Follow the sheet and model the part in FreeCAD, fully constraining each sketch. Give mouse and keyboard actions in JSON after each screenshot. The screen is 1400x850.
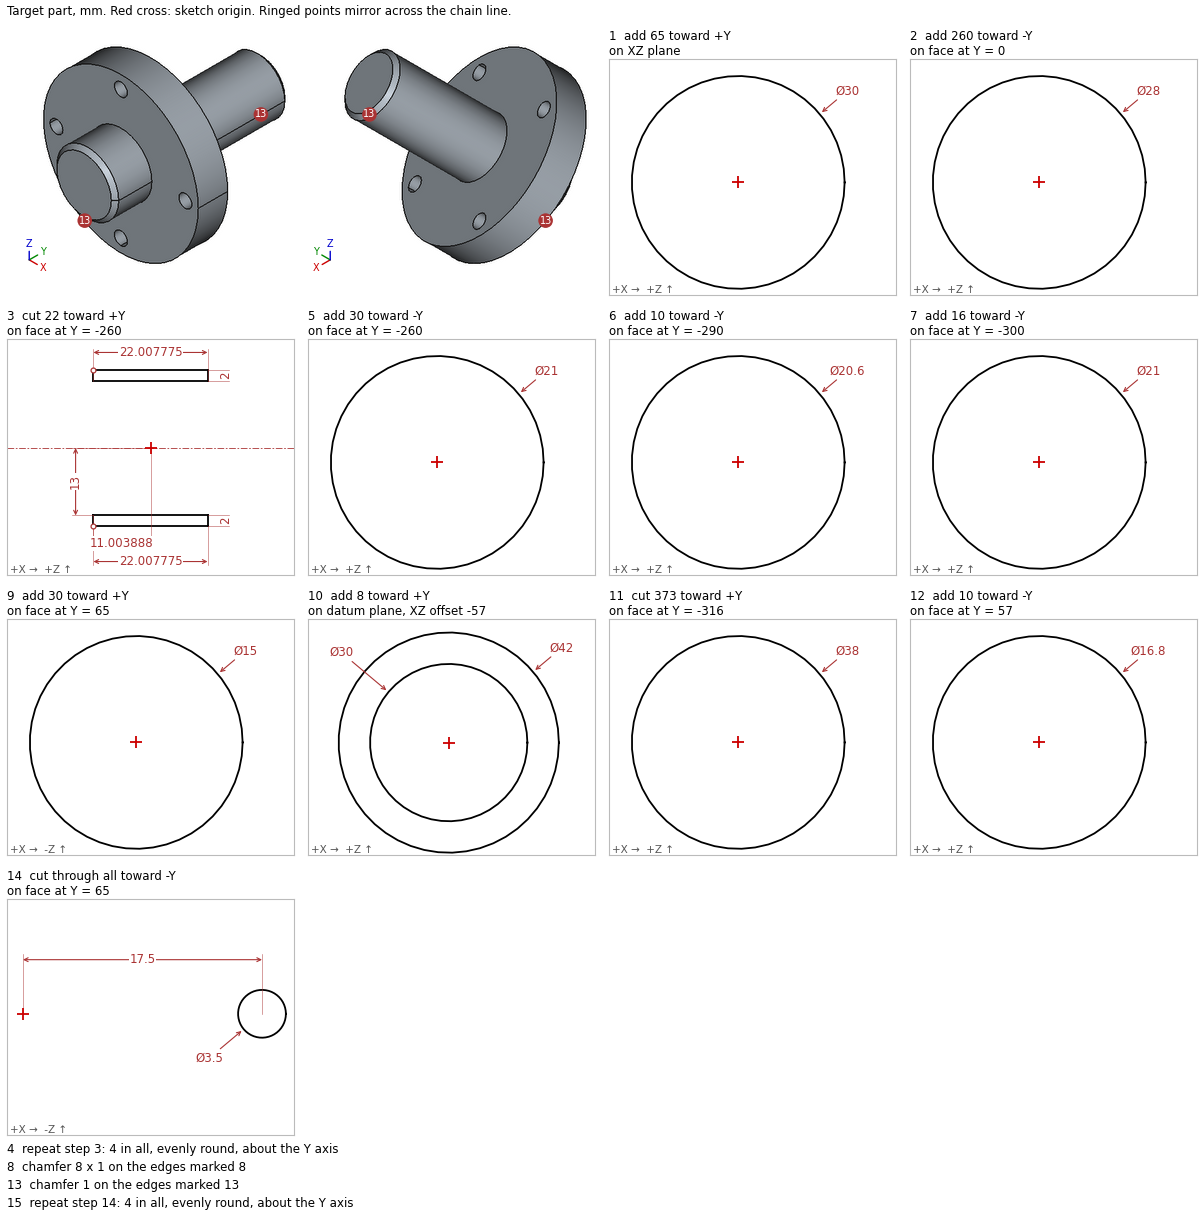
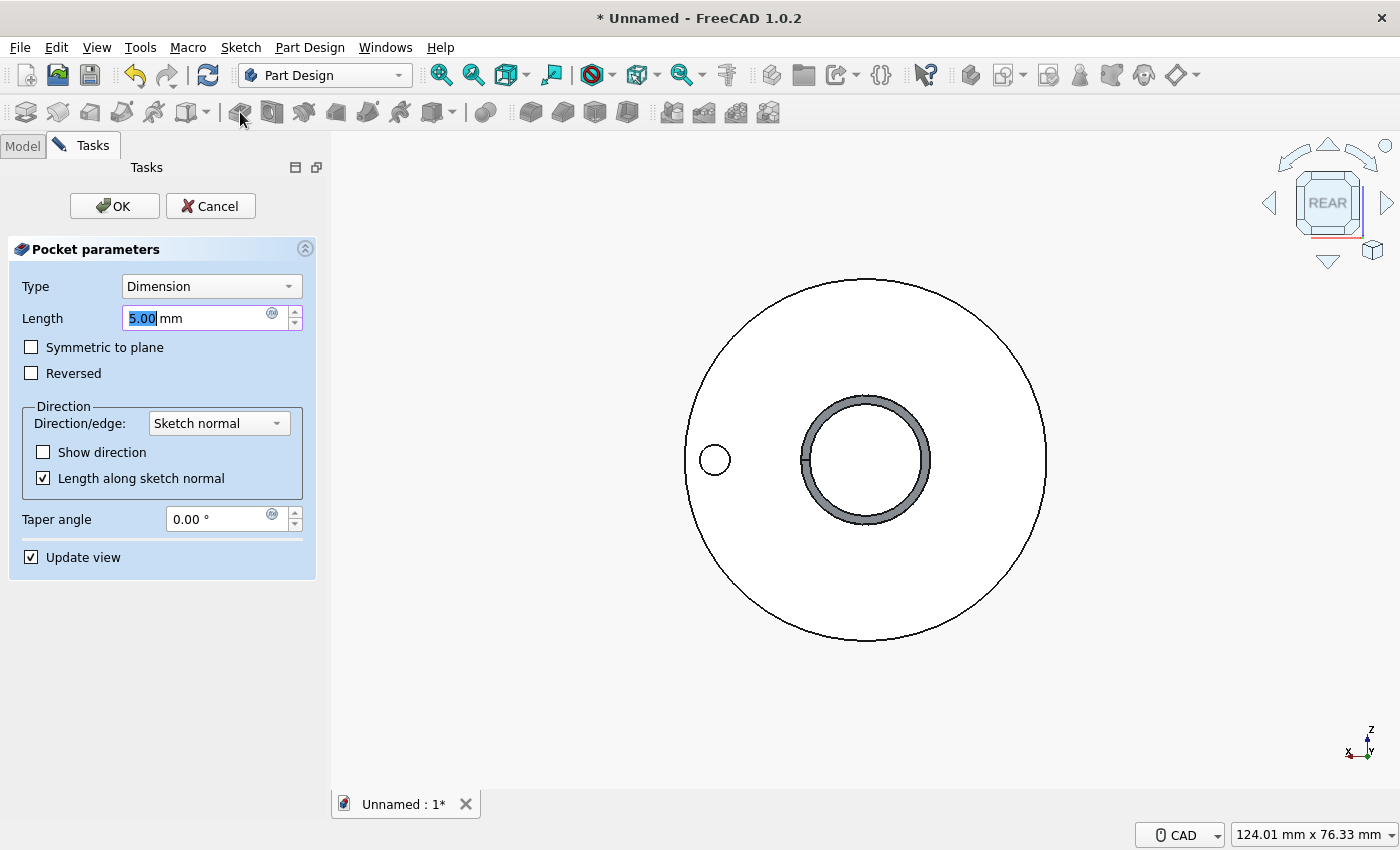
{"action": "left_click", "coordinate": [212, 286]}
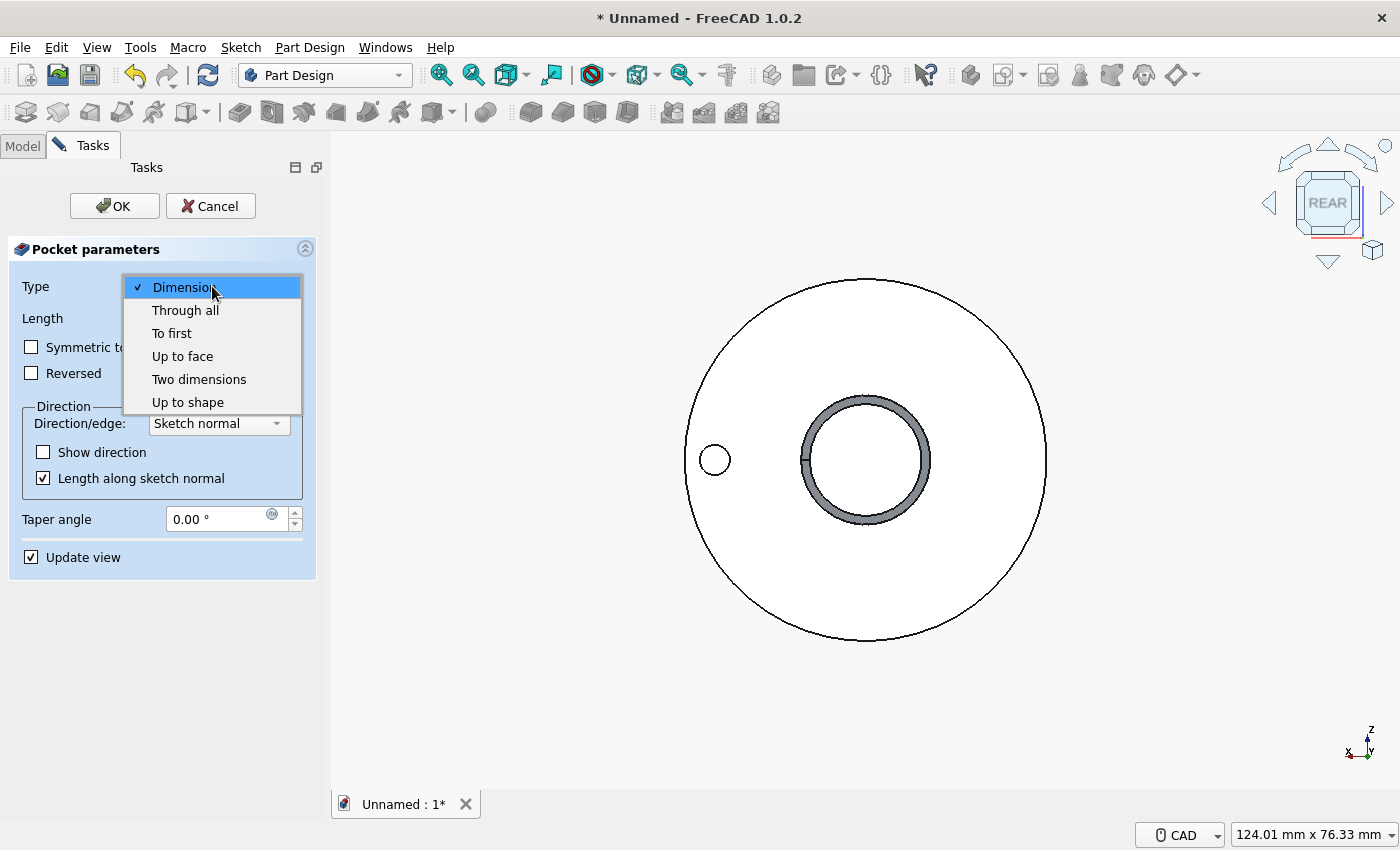
{"action": "left_click", "coordinate": [212, 310]}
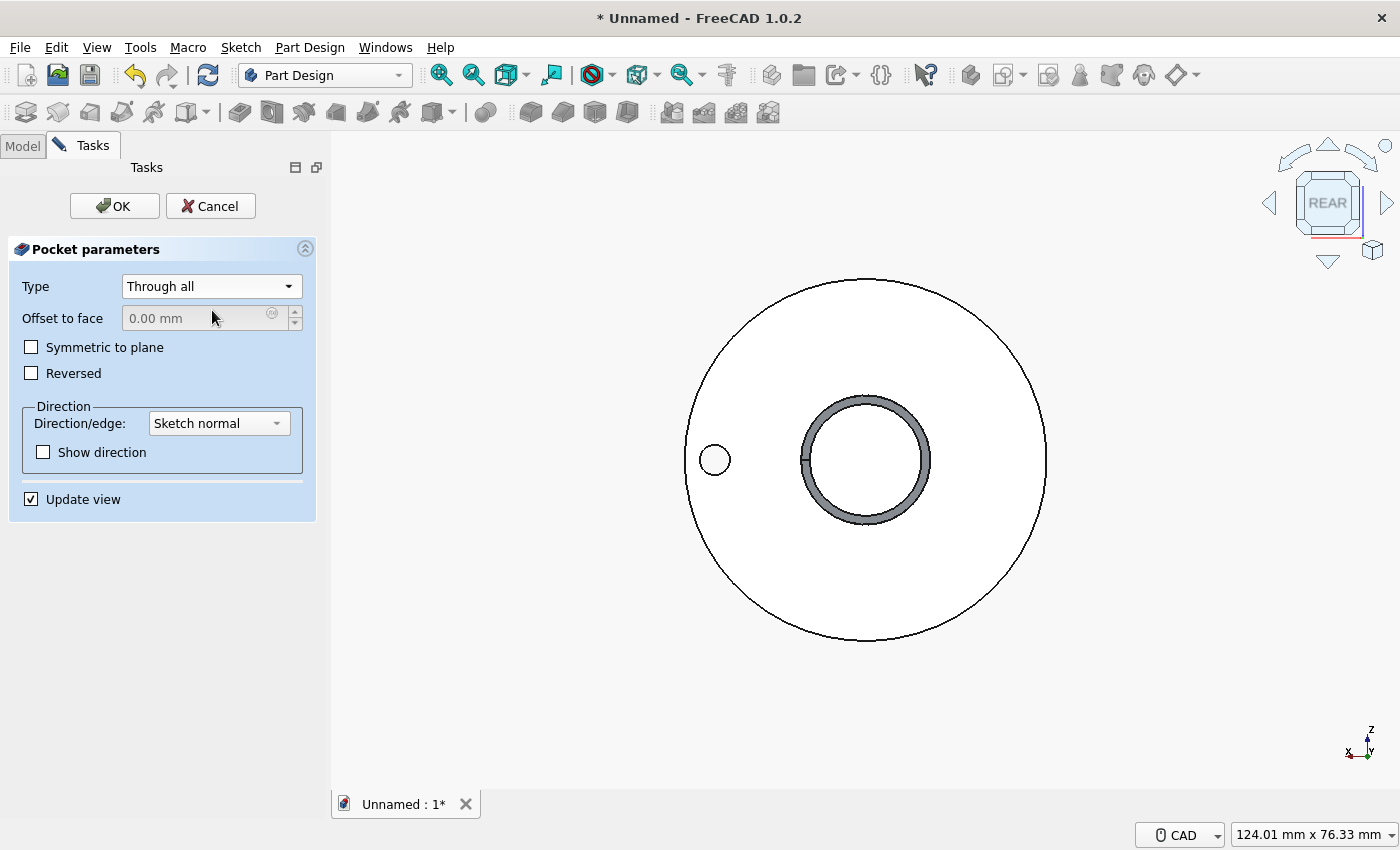
{"action": "left_click", "coordinate": [115, 206]}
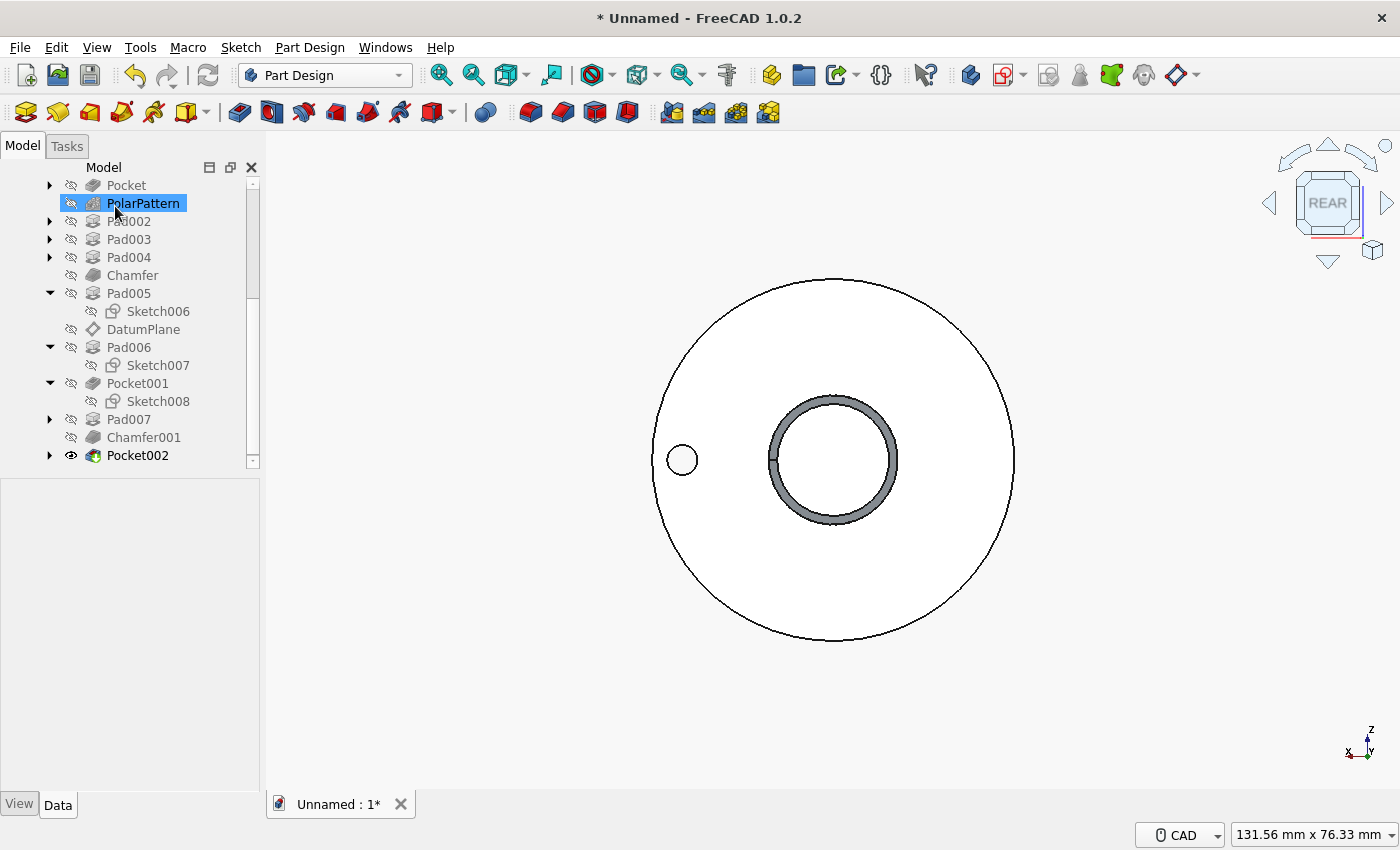
{"action": "left_click", "coordinate": [116, 455]}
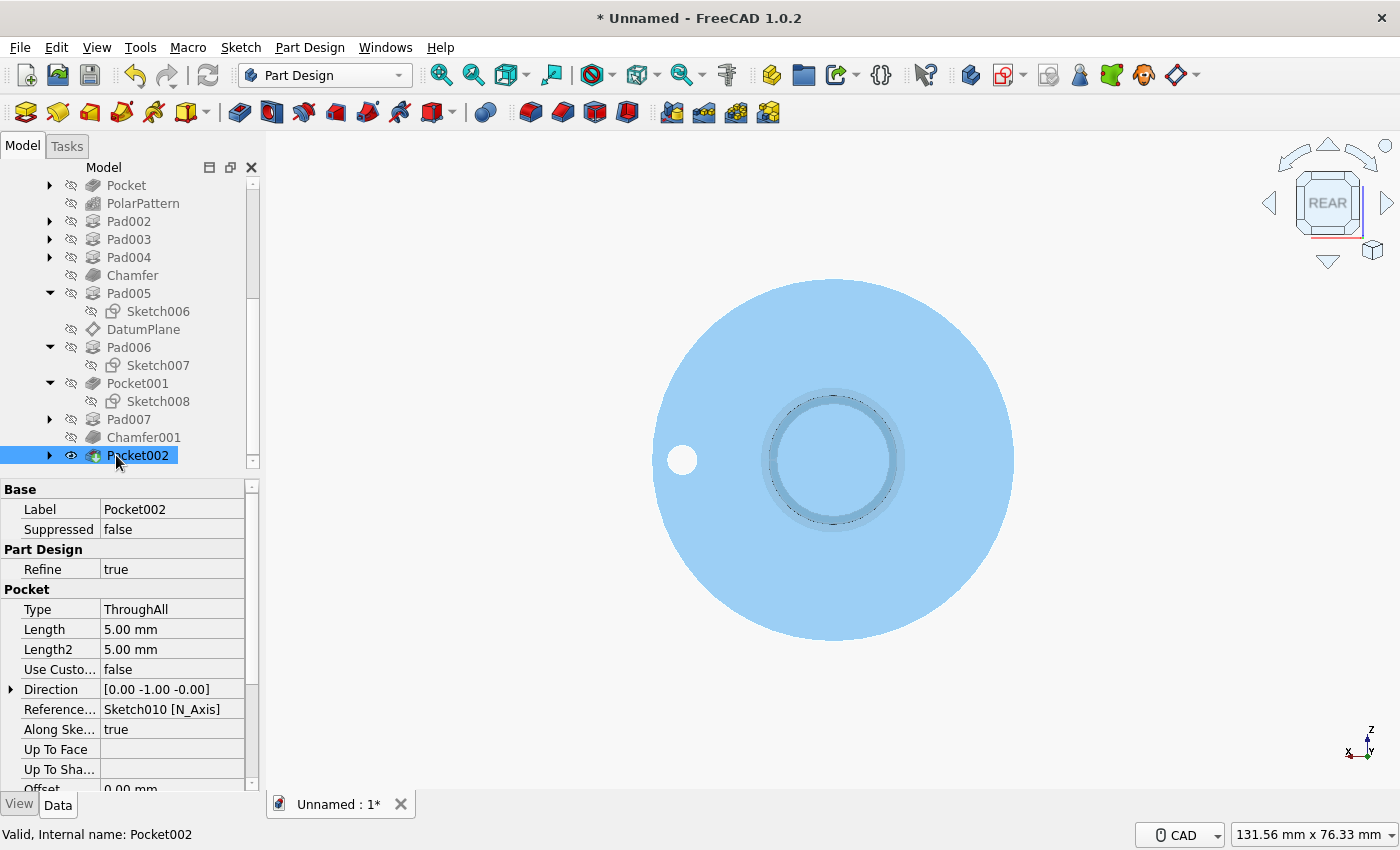
{"action": "left_click", "coordinate": [736, 112]}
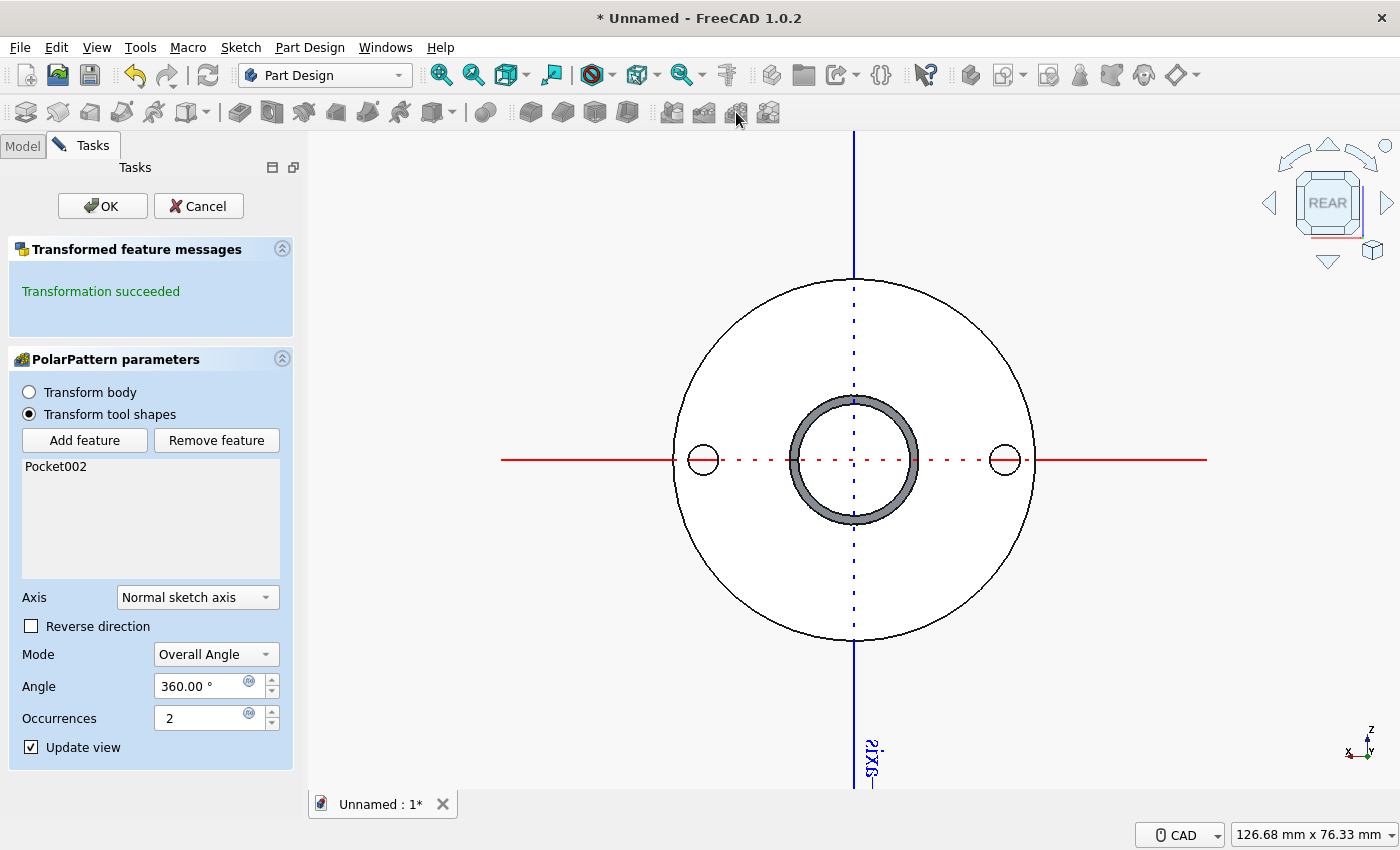
{"action": "left_click", "coordinate": [198, 598]}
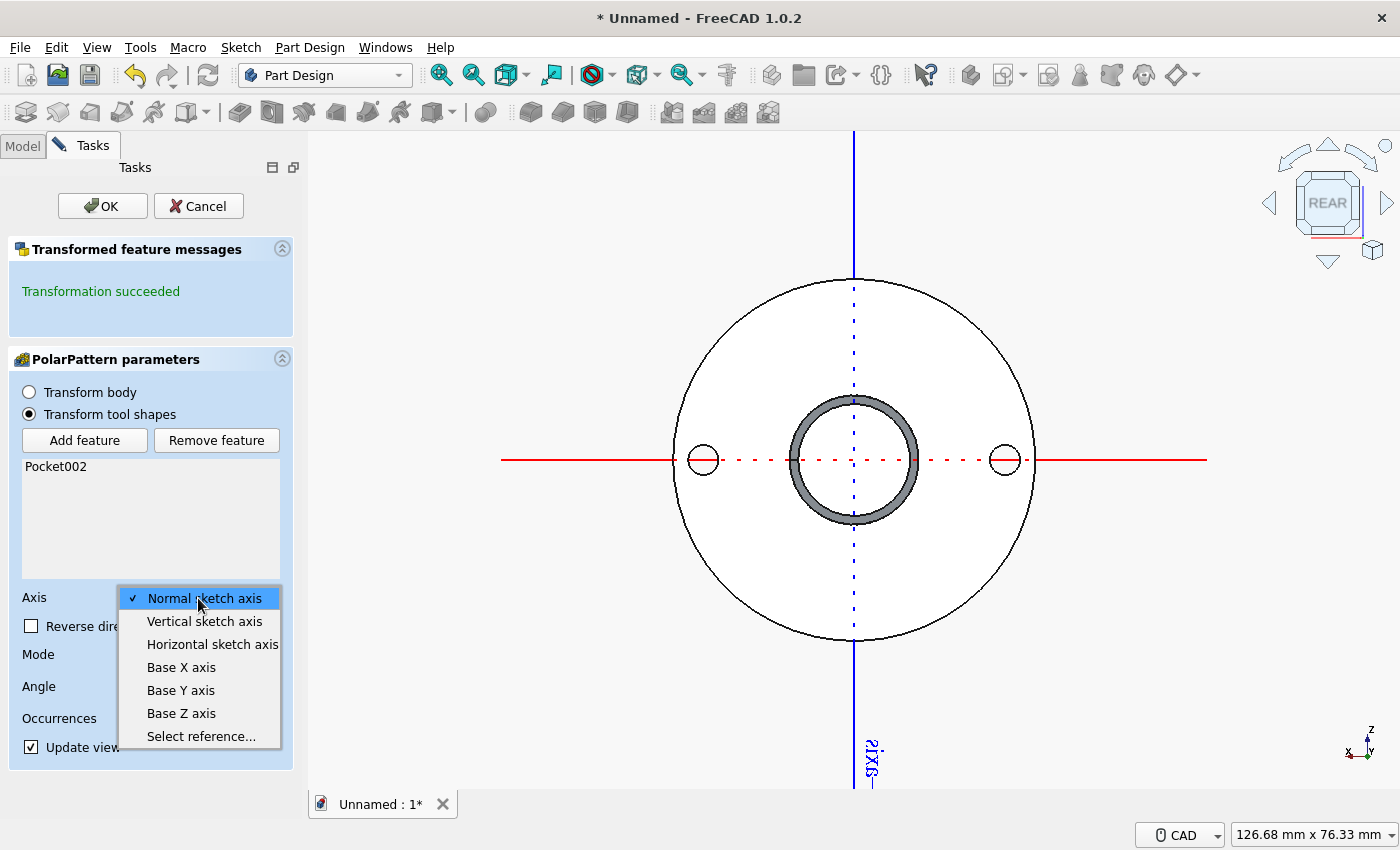
{"action": "left_click", "coordinate": [198, 690]}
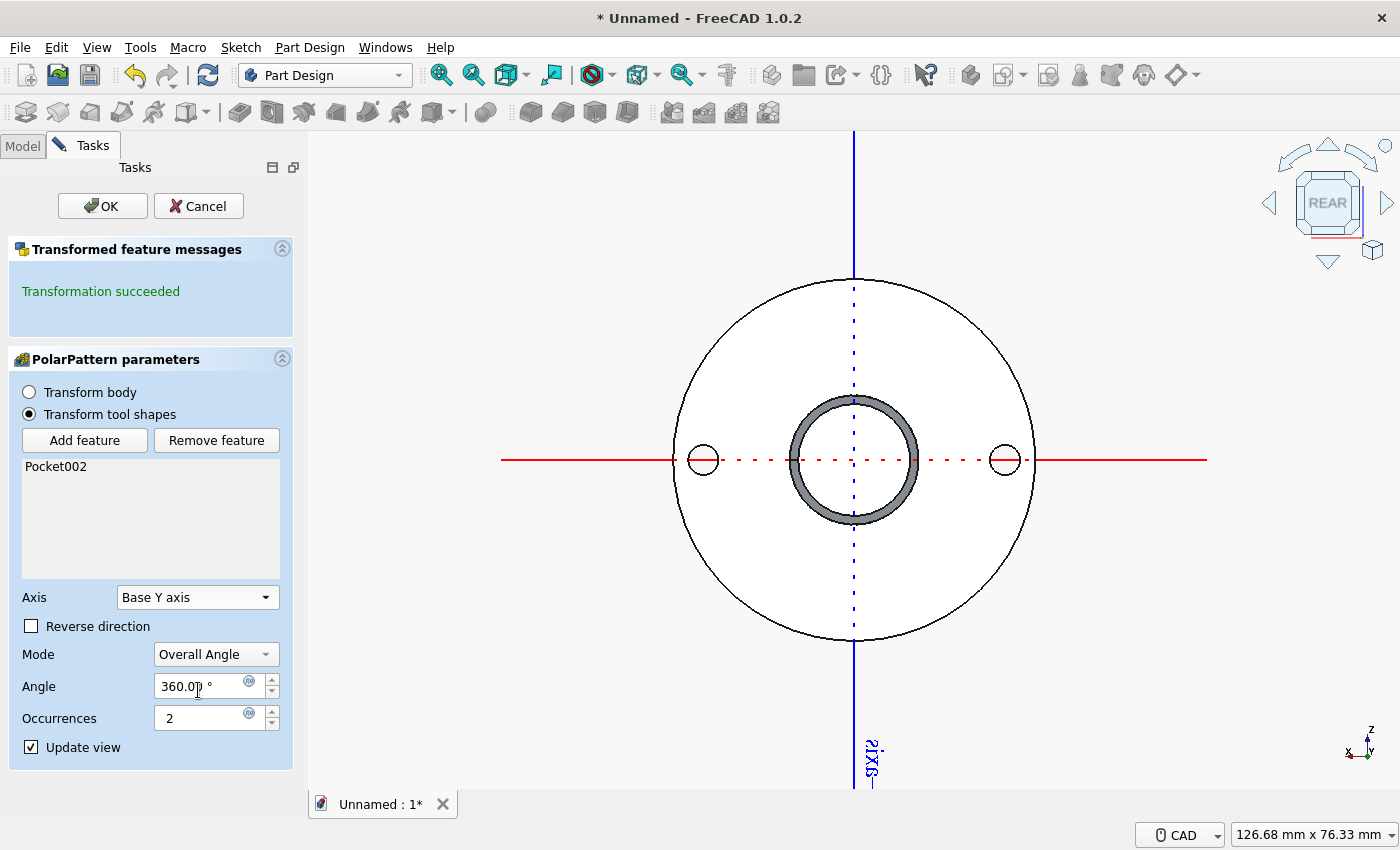
{"action": "triple_click", "coordinate": [209, 718]}